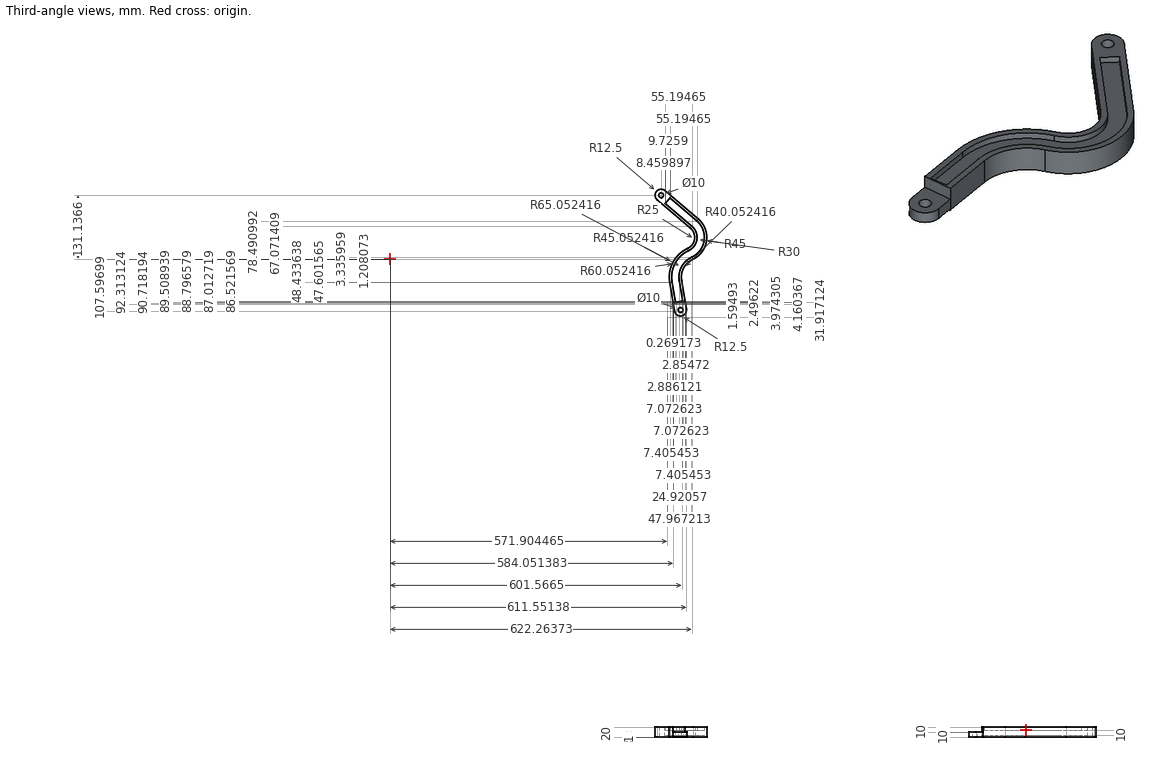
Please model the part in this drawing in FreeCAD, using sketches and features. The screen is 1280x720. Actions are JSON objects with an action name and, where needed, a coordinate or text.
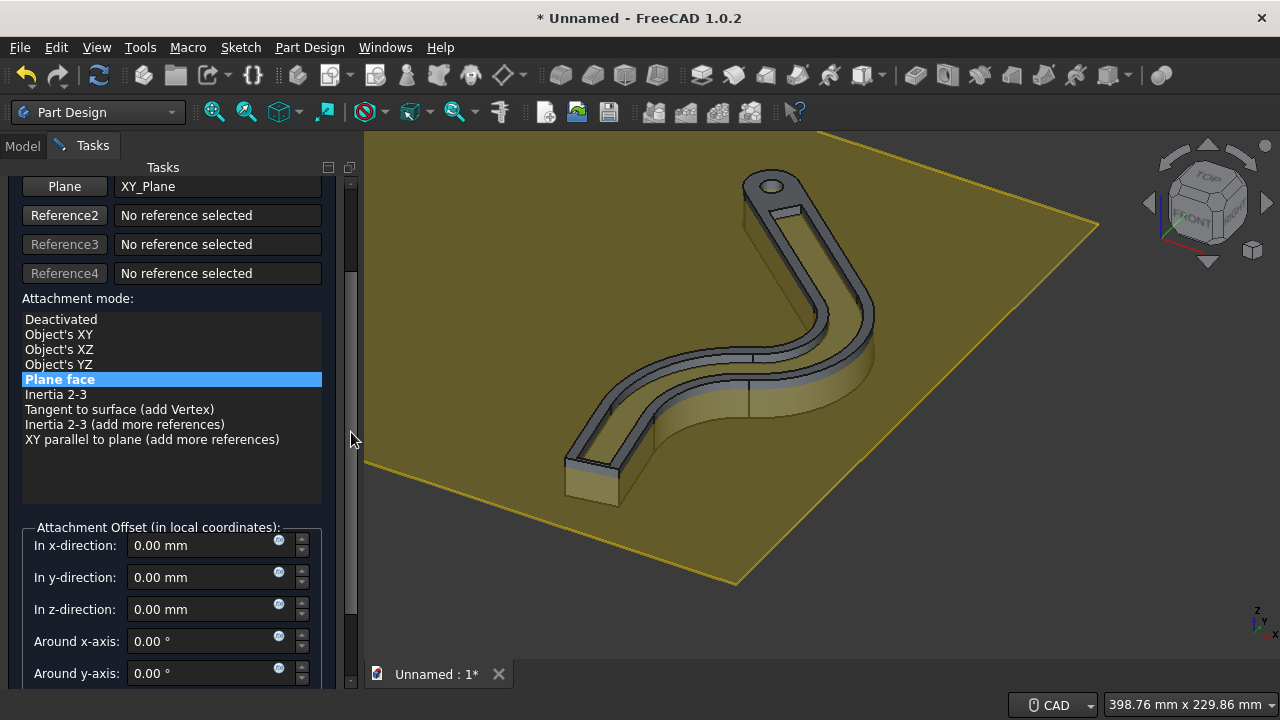
{"action": "triple_click", "coordinate": [210, 609]}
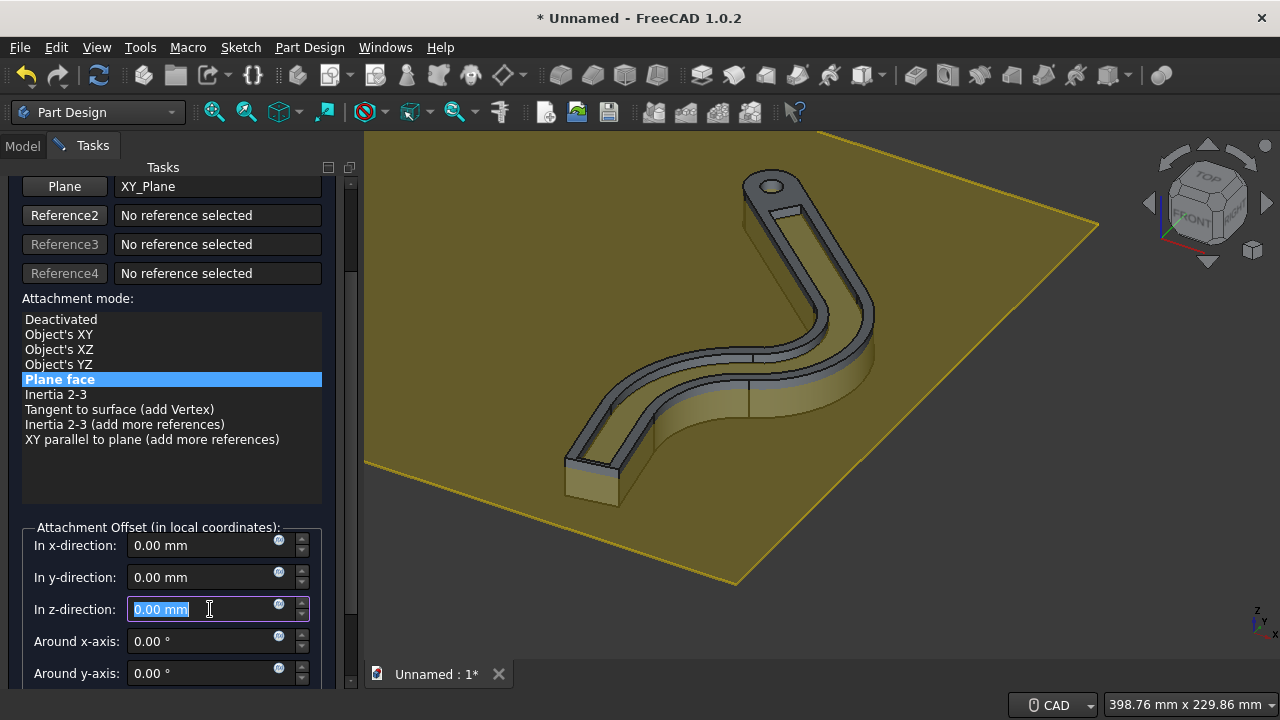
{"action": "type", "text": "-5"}
{"action": "key", "text": "Tab"}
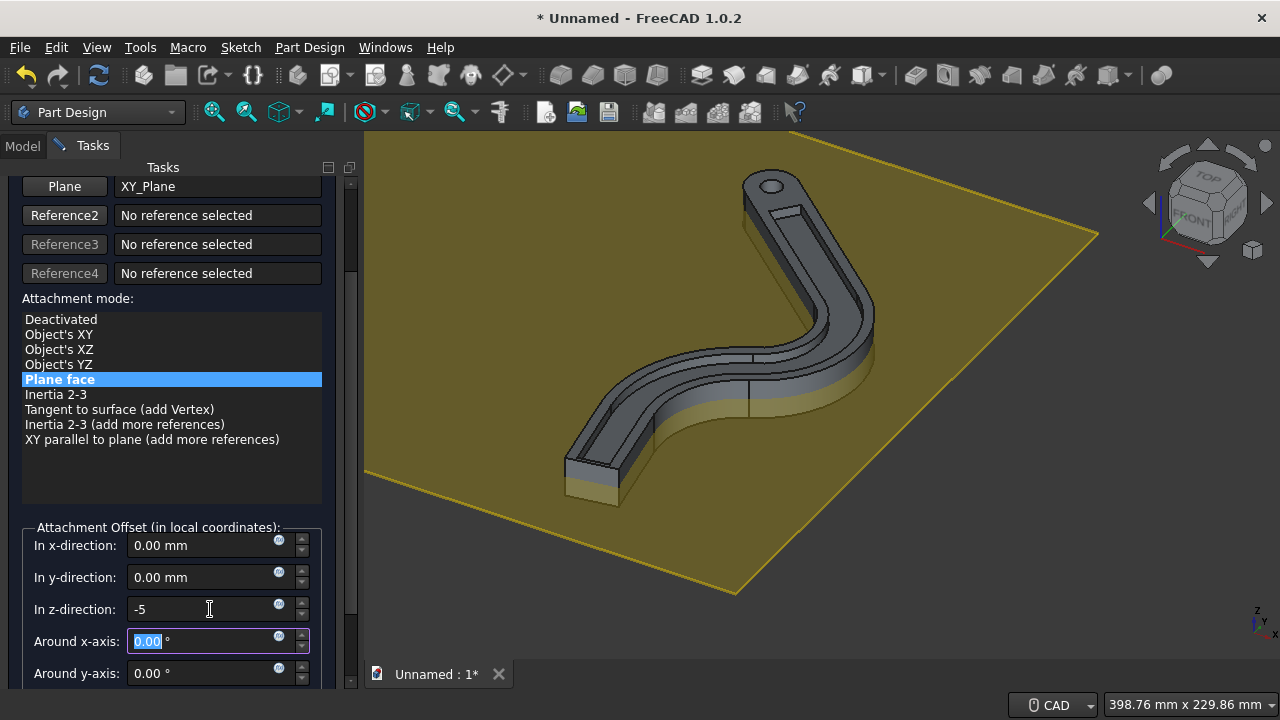
{"action": "scroll", "coordinate": [351, 432], "scroll_direction": "up", "scroll_amount": 3}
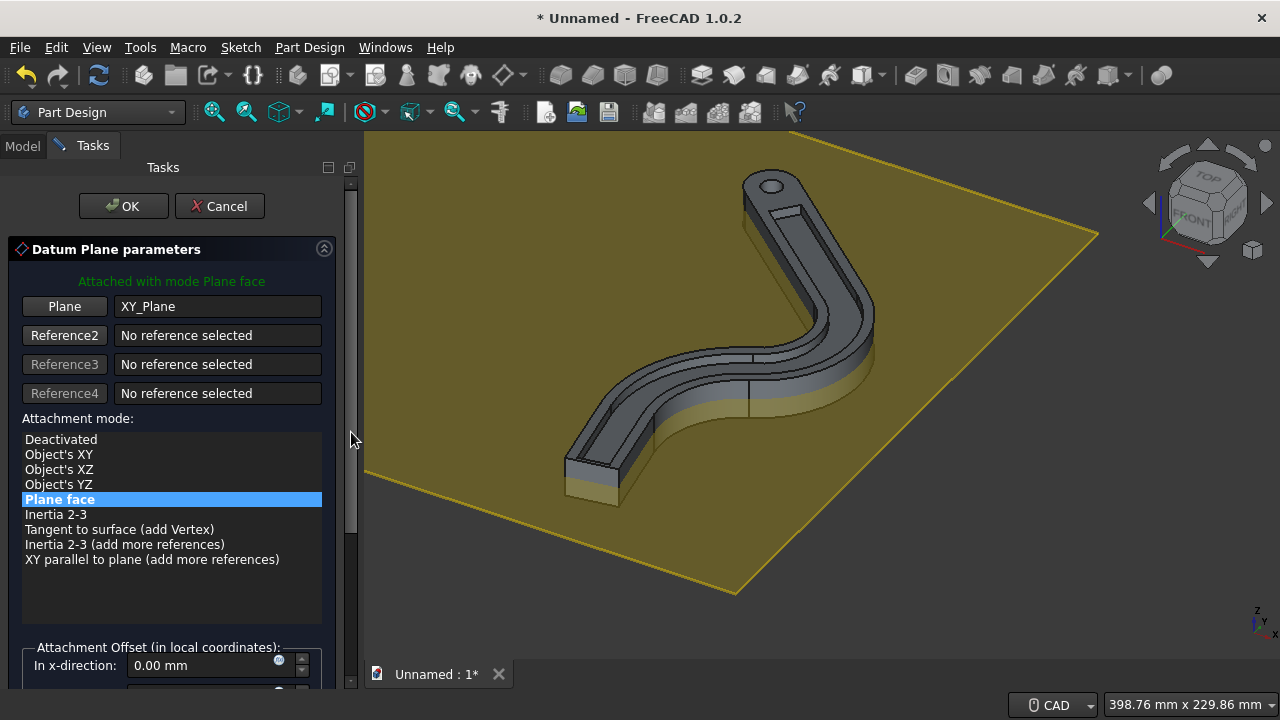
{"action": "left_click", "coordinate": [124, 206]}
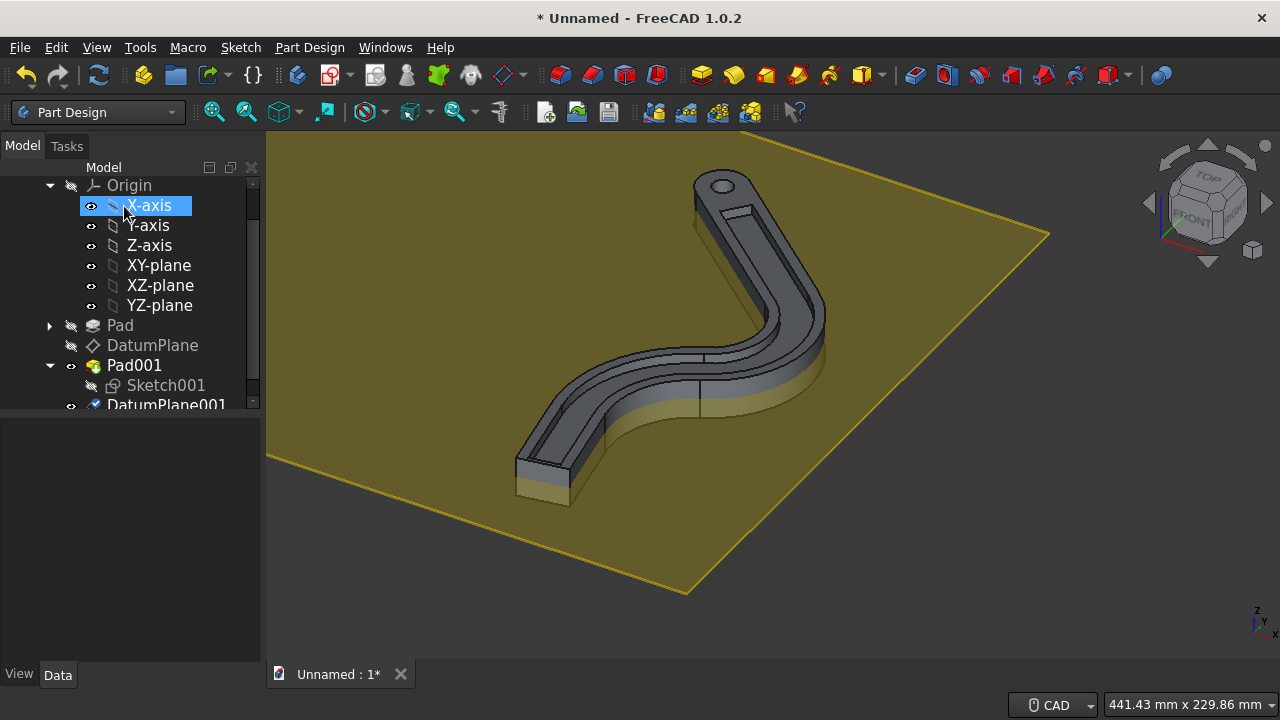
{"action": "left_click", "coordinate": [116, 406]}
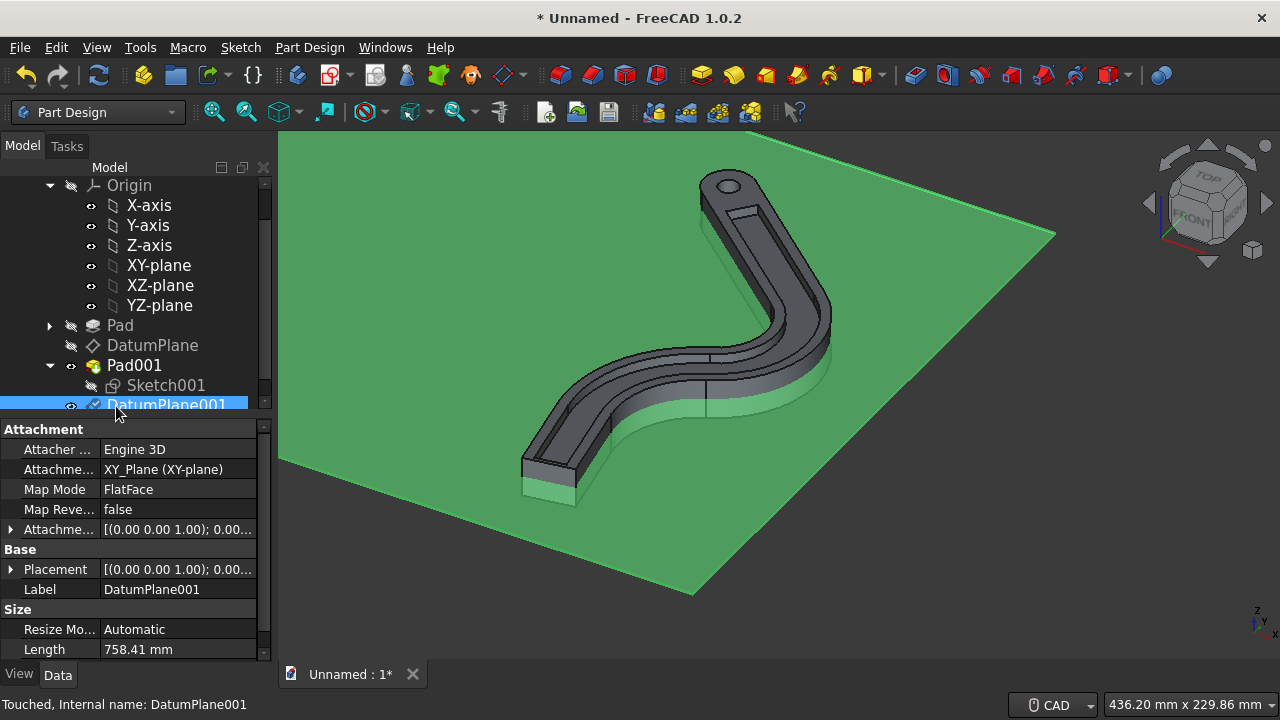
{"action": "left_click", "coordinate": [330, 76]}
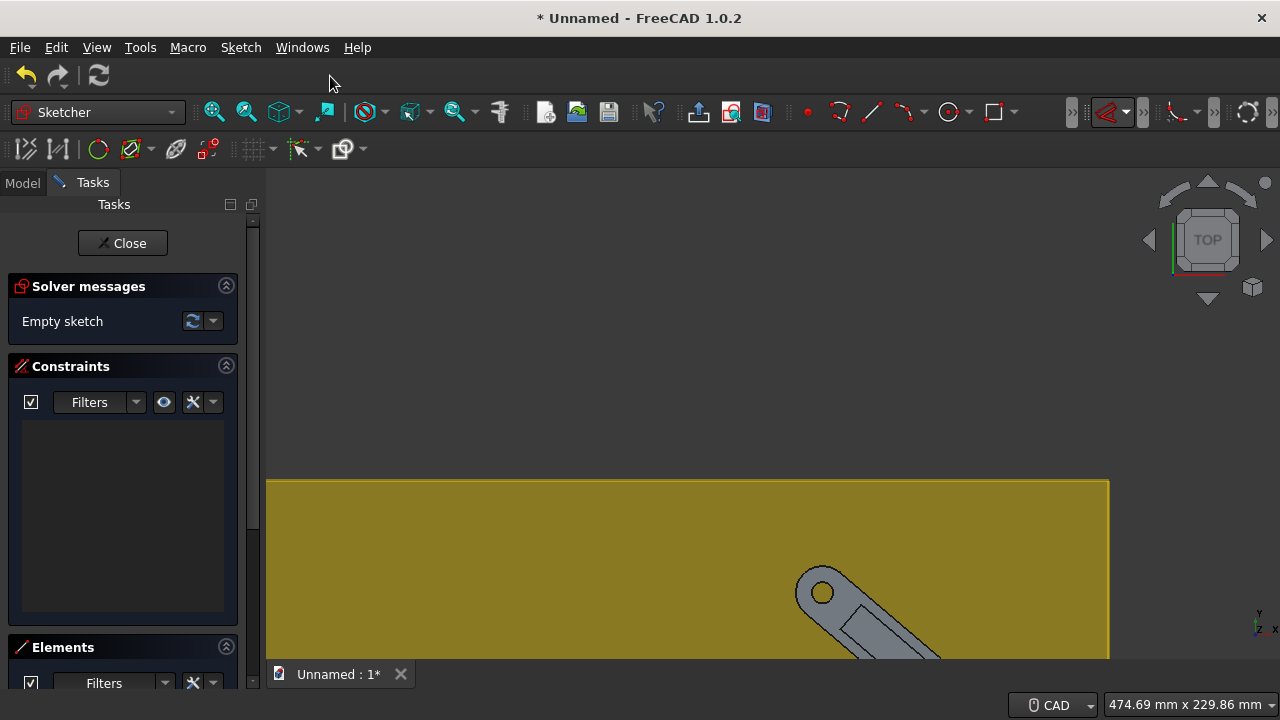
{"action": "left_click", "coordinate": [764, 112]}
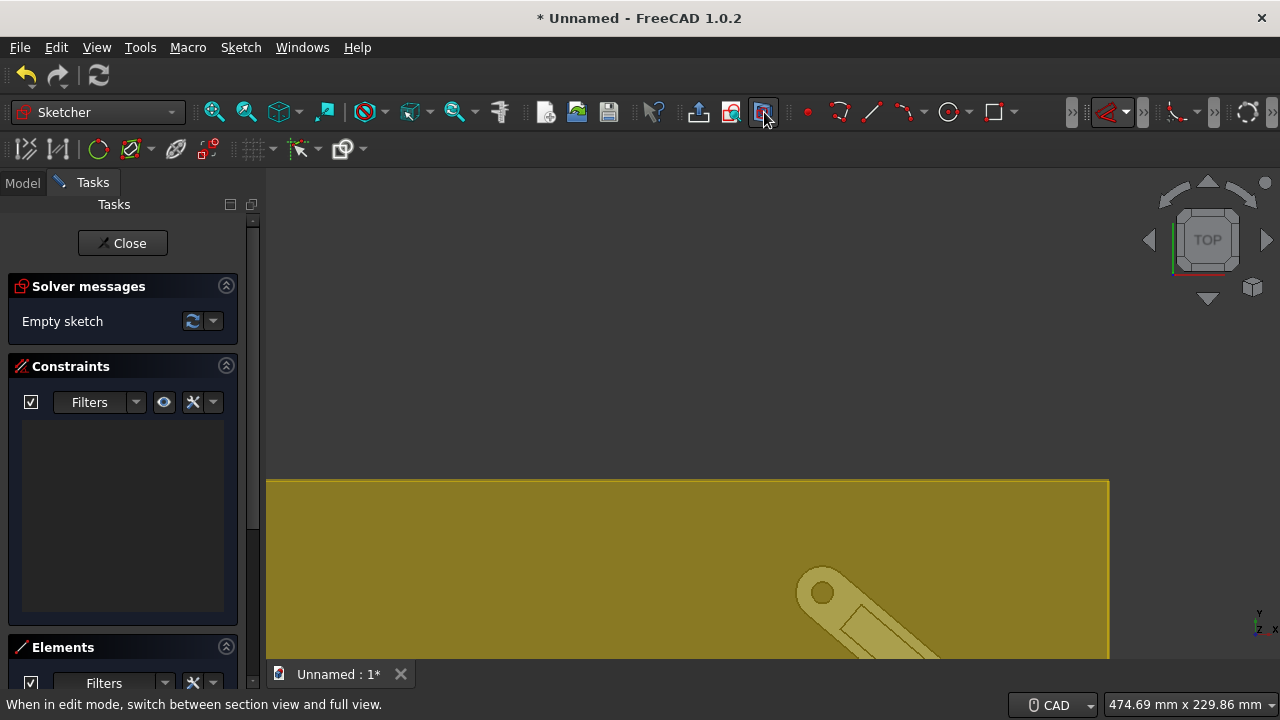
{"action": "scroll", "coordinate": [704, 414], "scroll_direction": "down", "scroll_amount": 5}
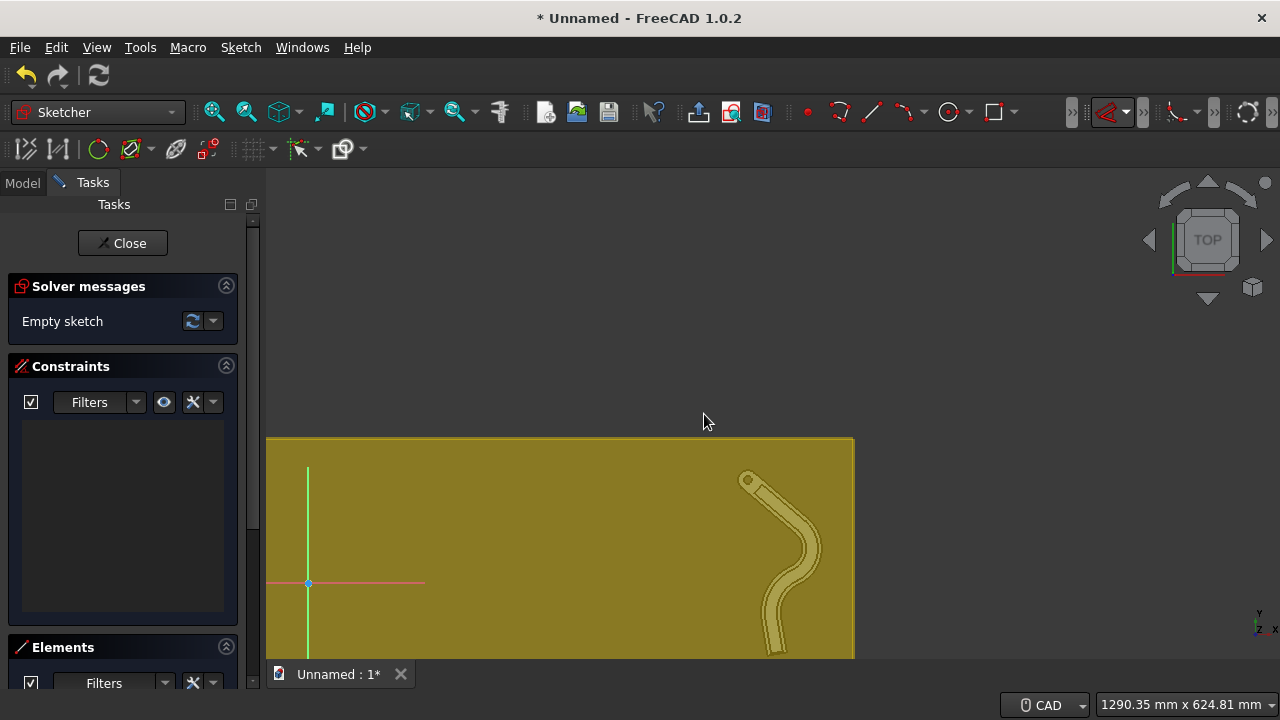
{"action": "scroll", "coordinate": [704, 414], "scroll_direction": "down", "scroll_amount": 5}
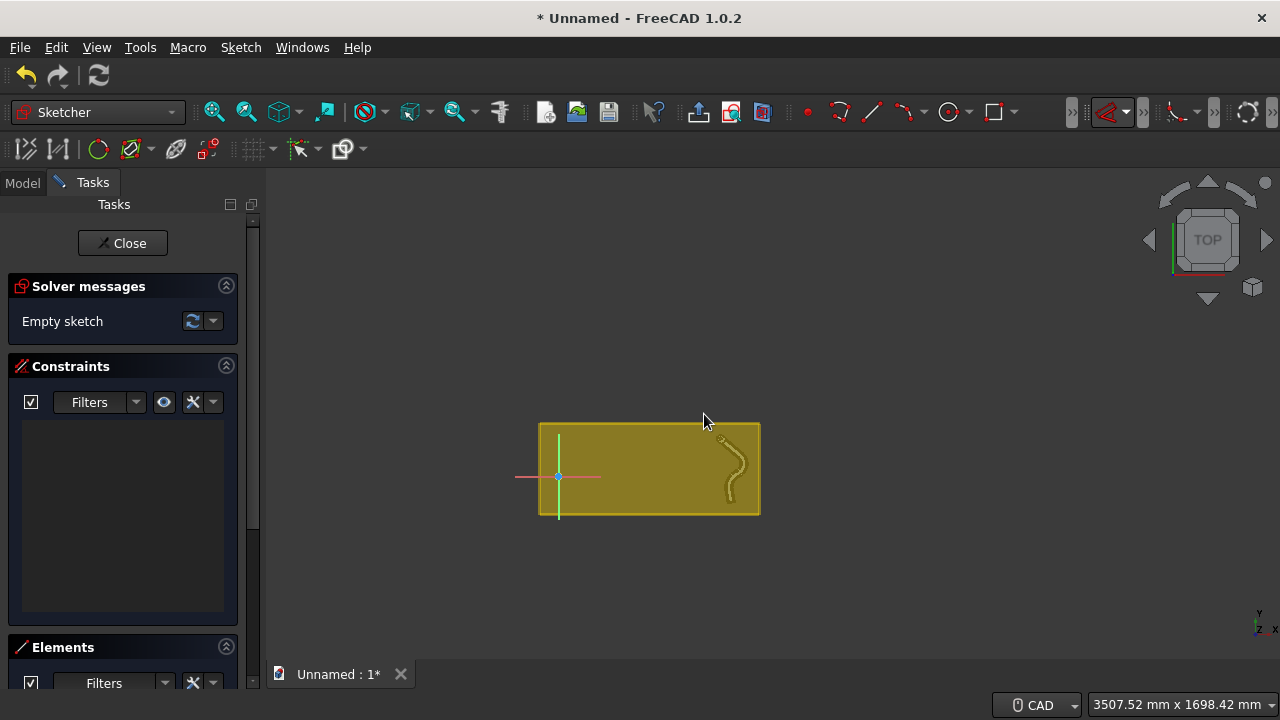
{"action": "scroll", "coordinate": [733, 511], "scroll_direction": "up", "scroll_amount": 15}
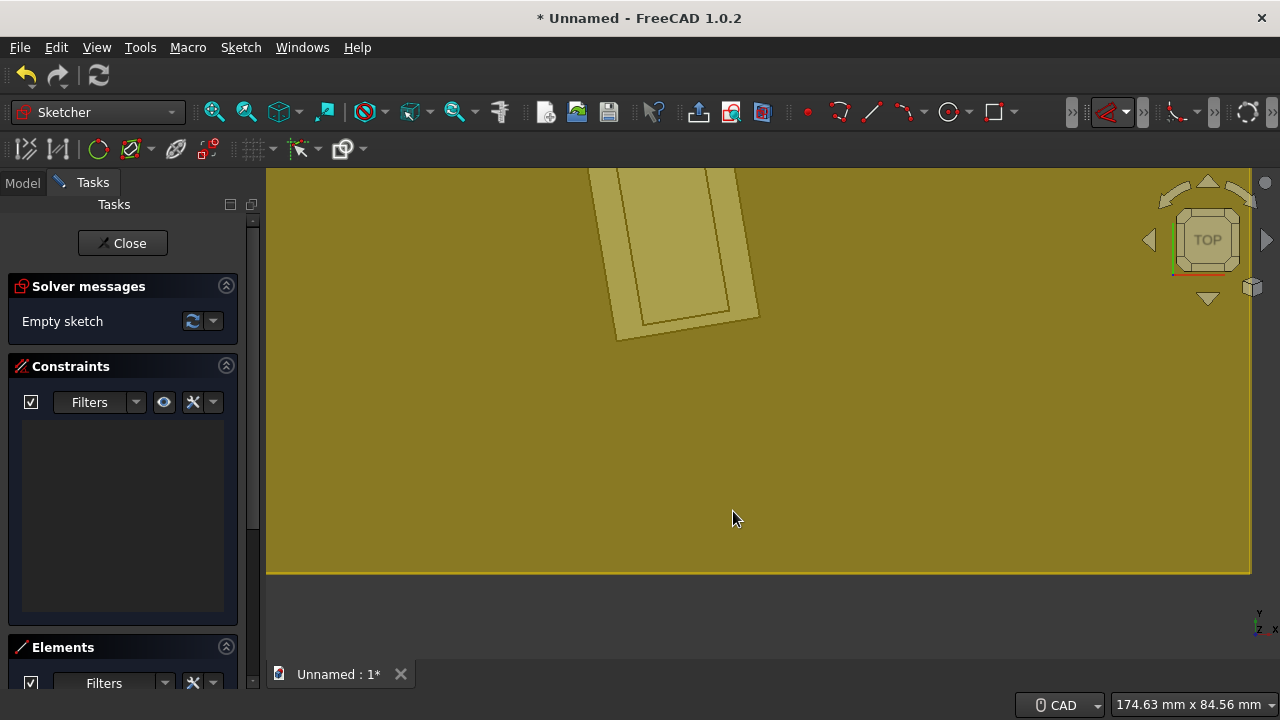
{"action": "scroll", "coordinate": [683, 381], "scroll_direction": "up", "scroll_amount": 3}